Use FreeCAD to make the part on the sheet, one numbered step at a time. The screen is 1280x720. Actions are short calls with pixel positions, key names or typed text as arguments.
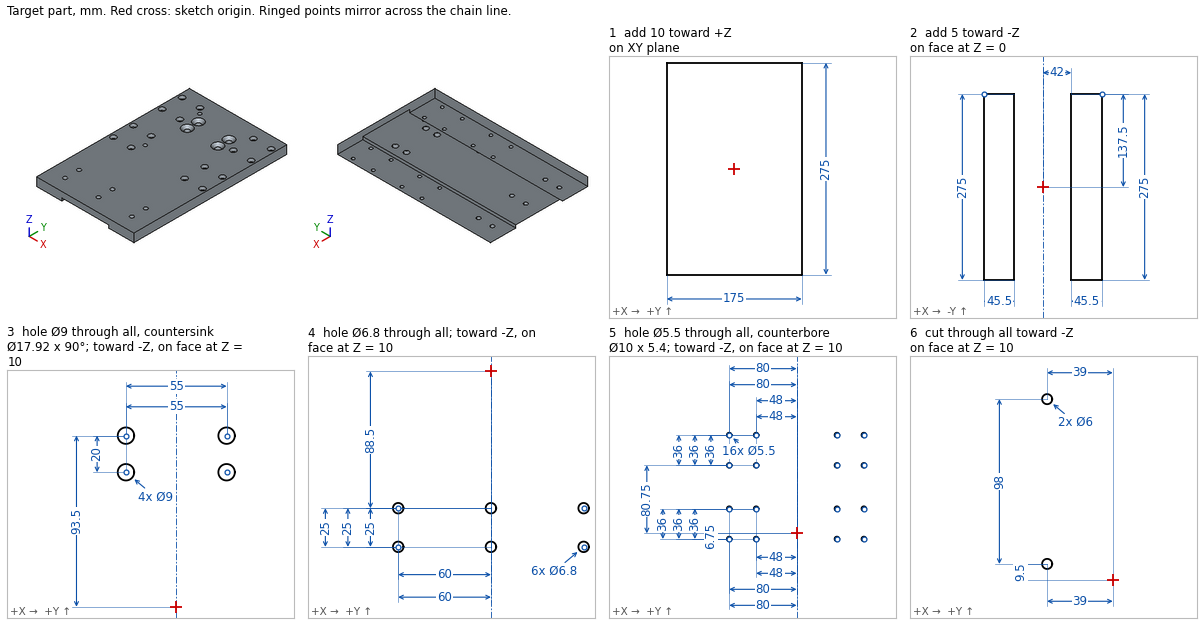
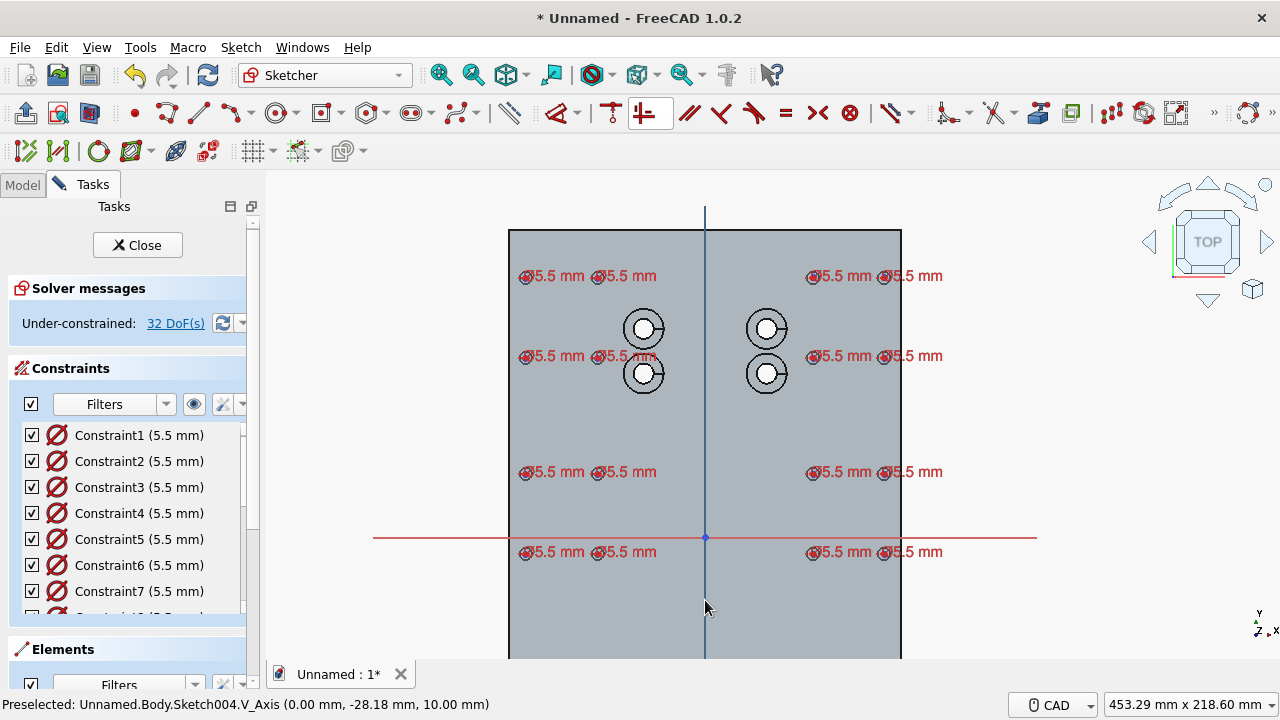
key(s)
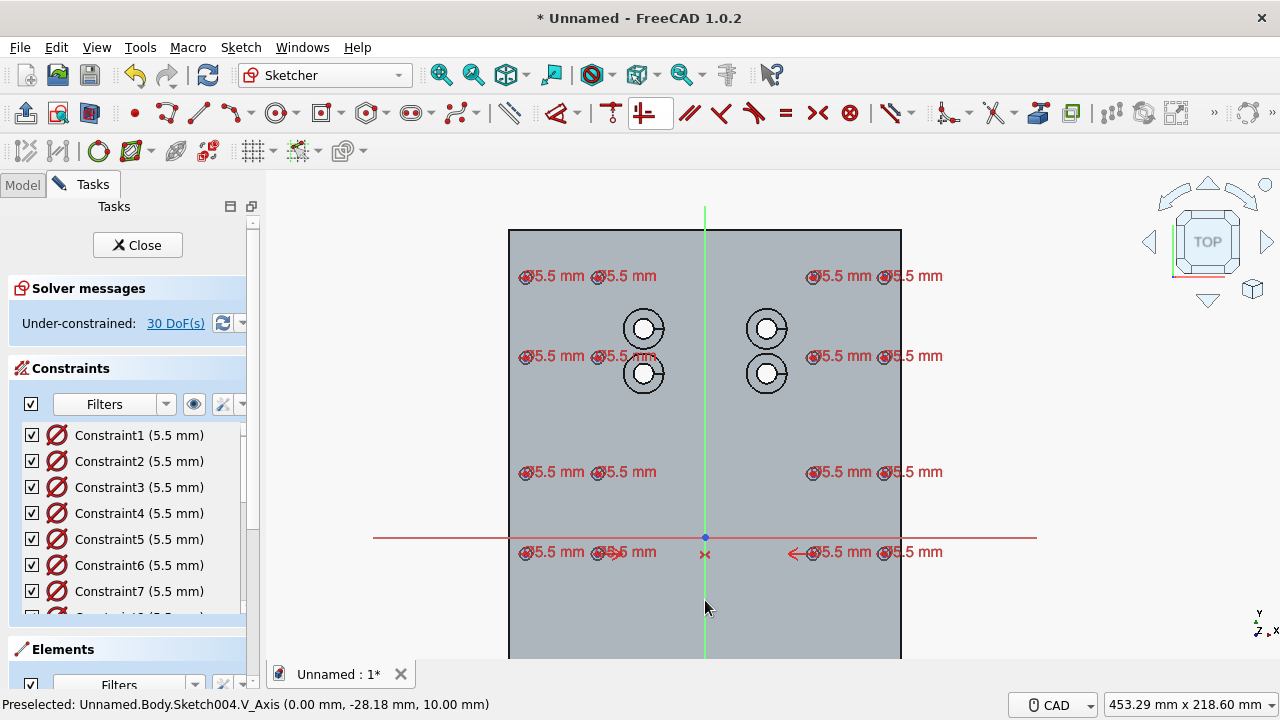
click(526, 554)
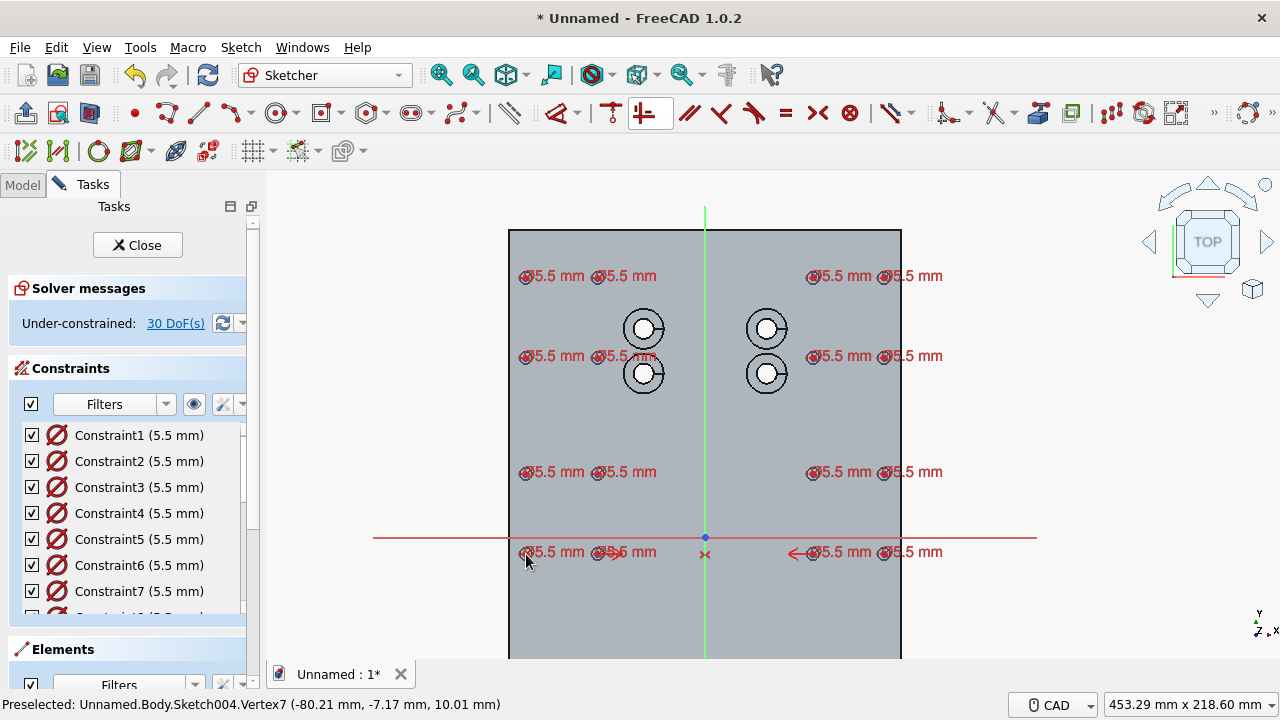
click(884, 554)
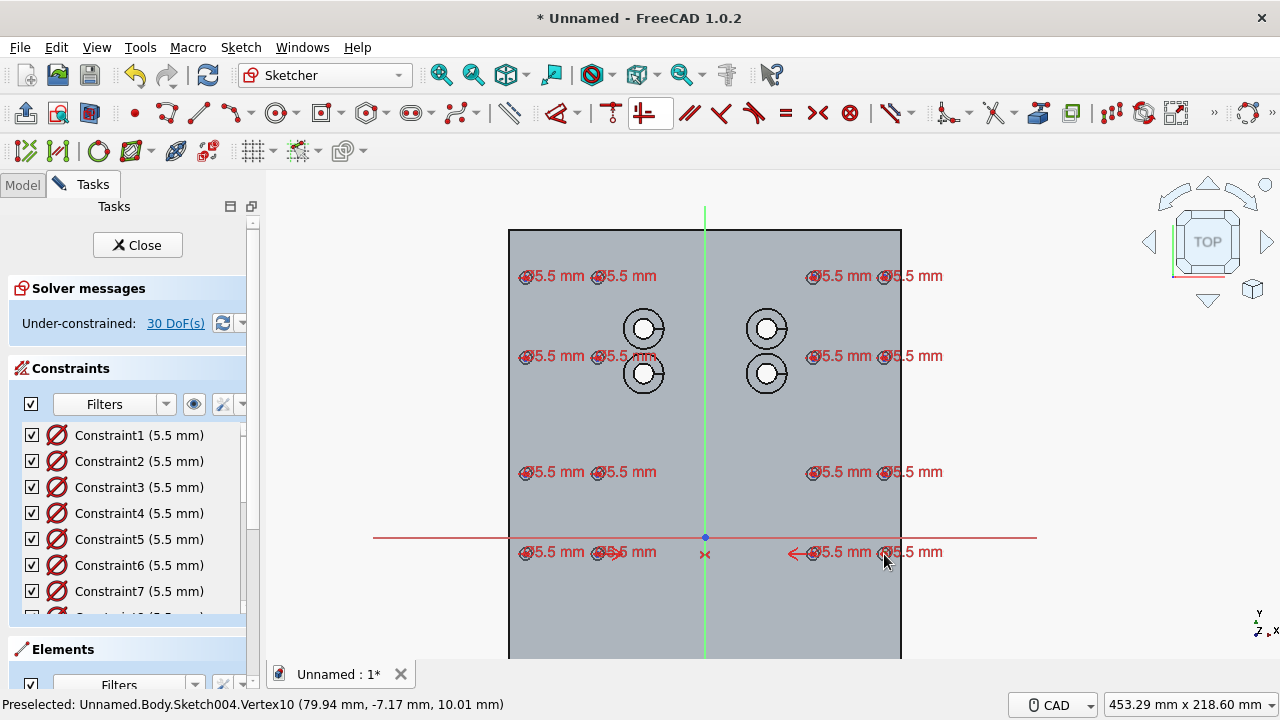
click(705, 600)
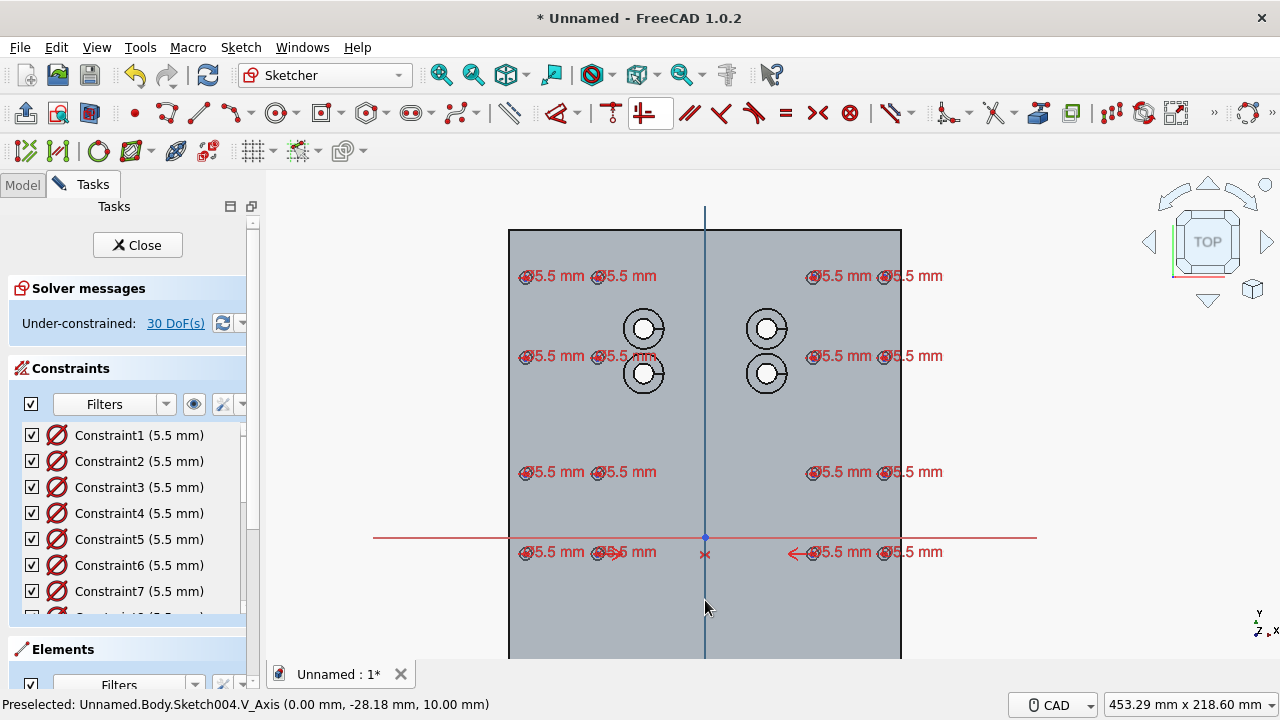
key(s)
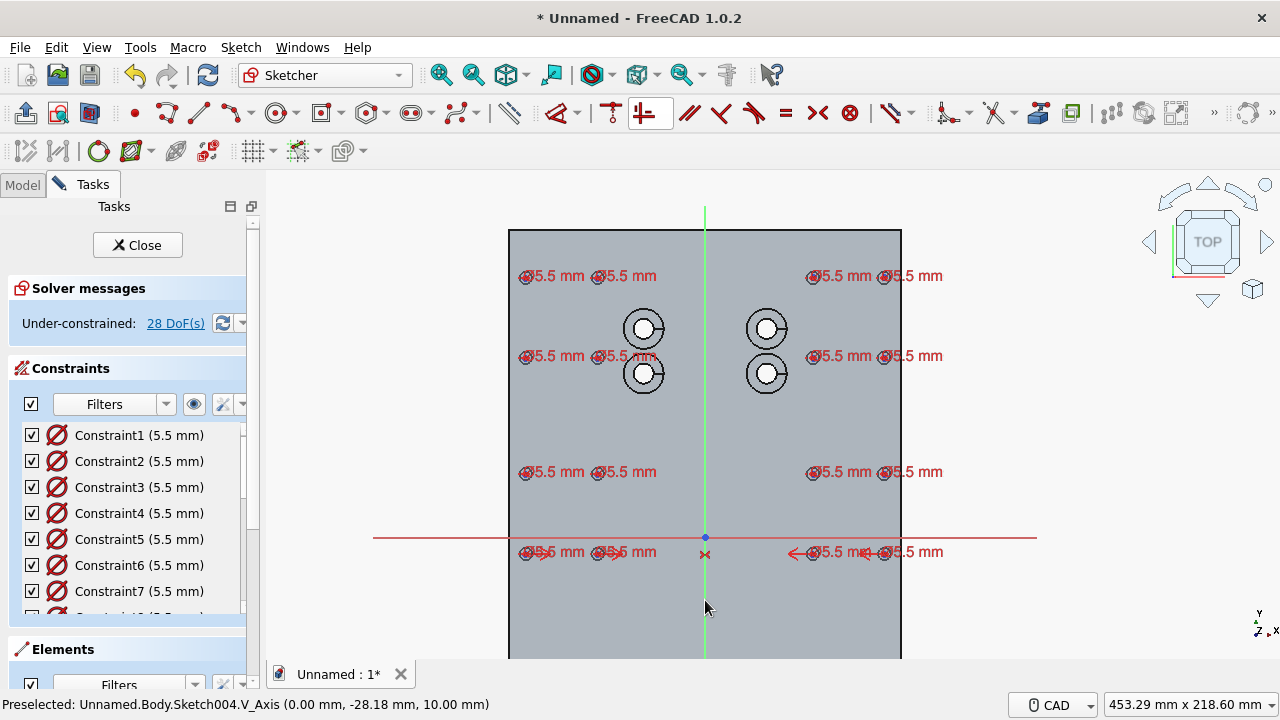
click(598, 474)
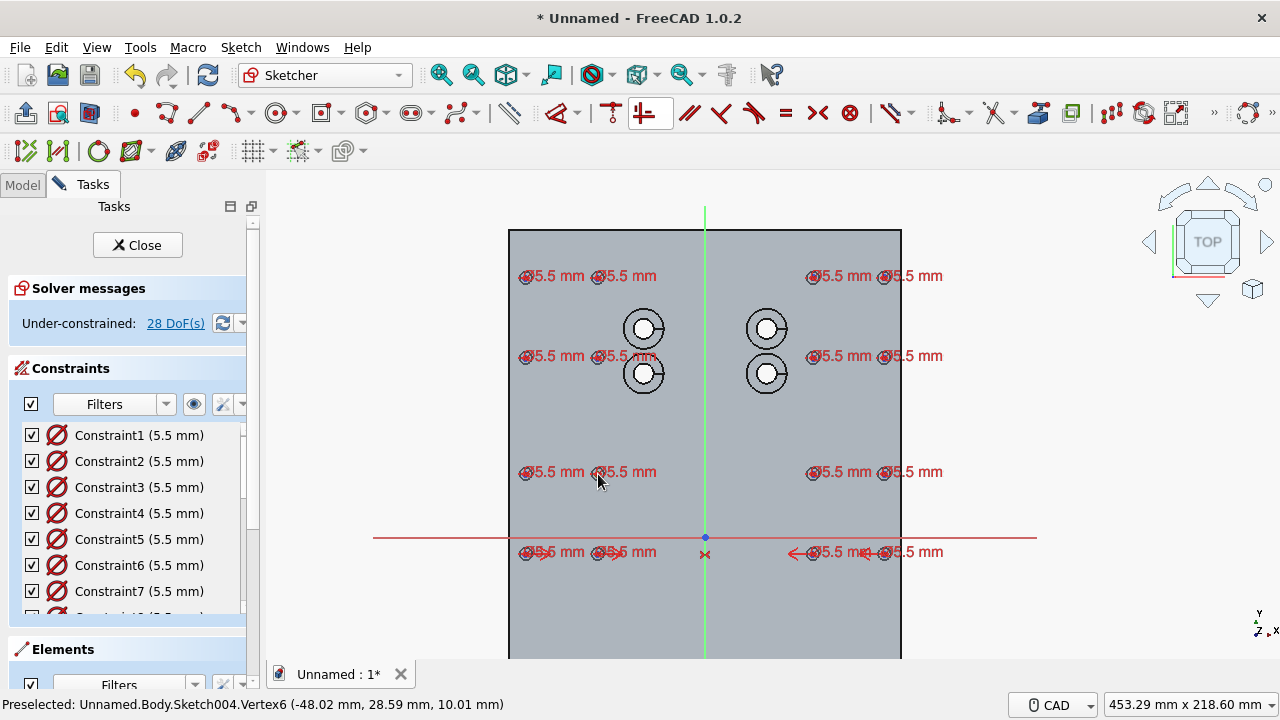
click(813, 474)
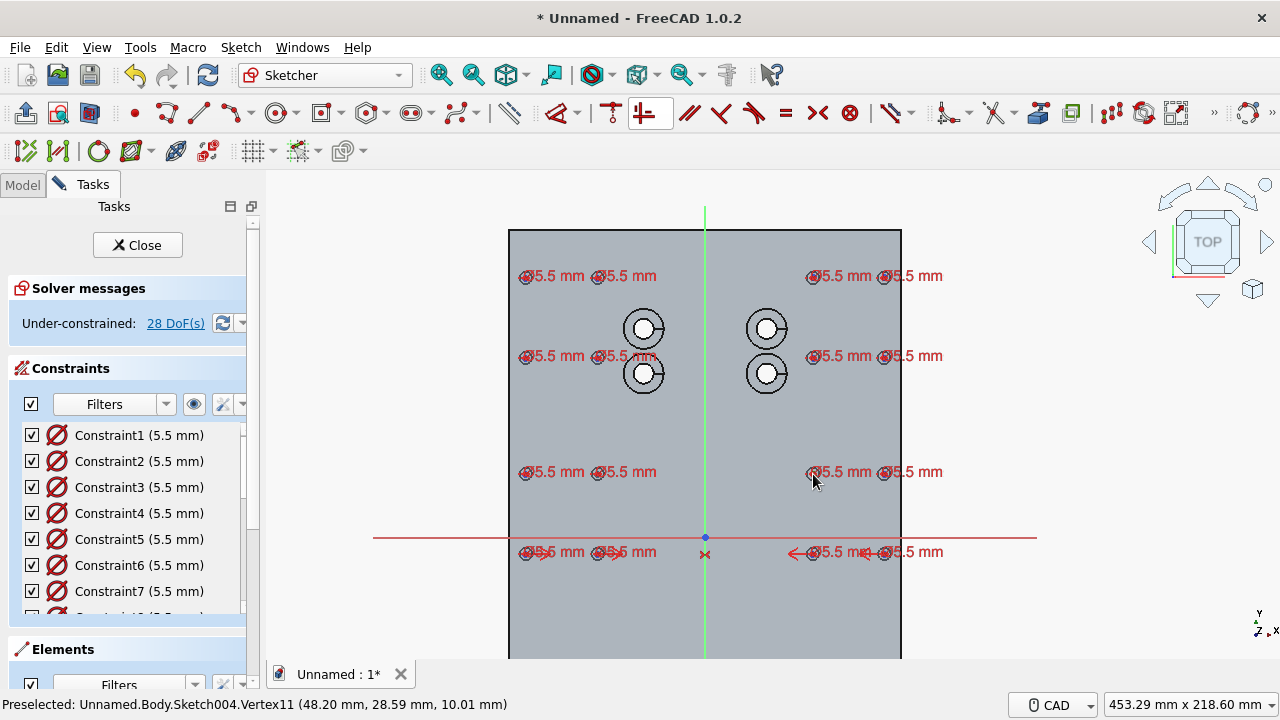
click(705, 600)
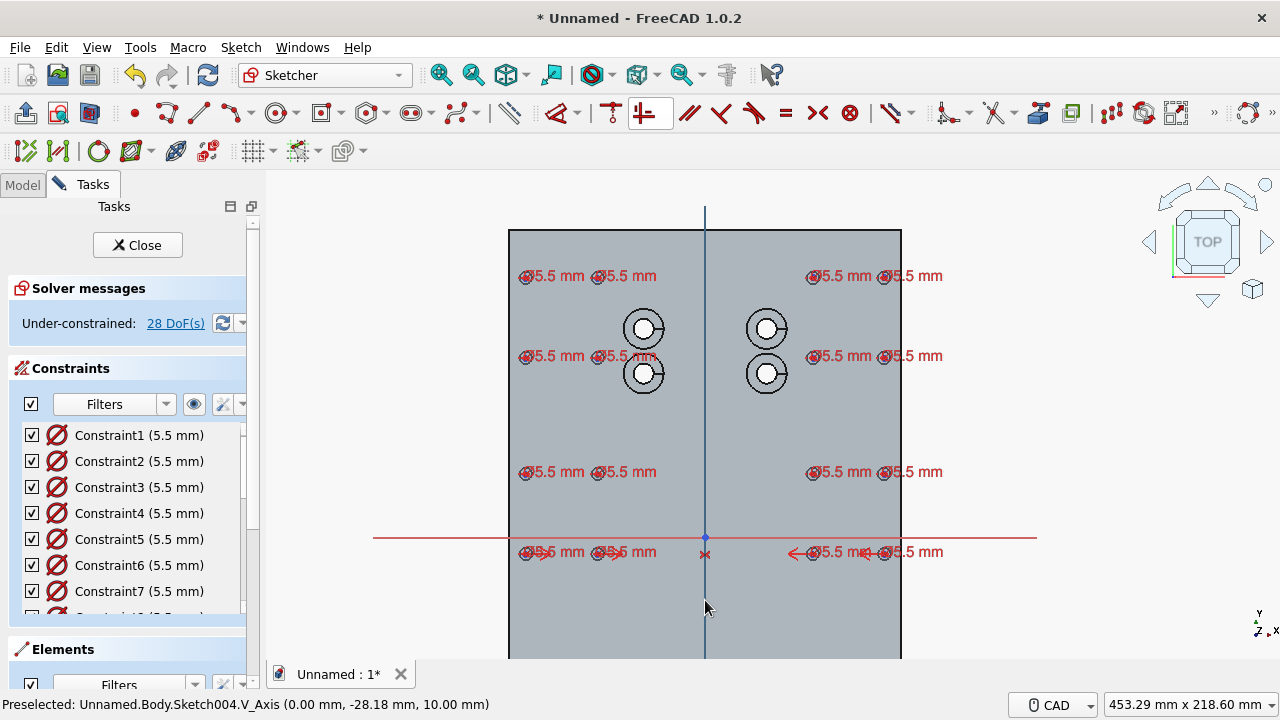
key(s)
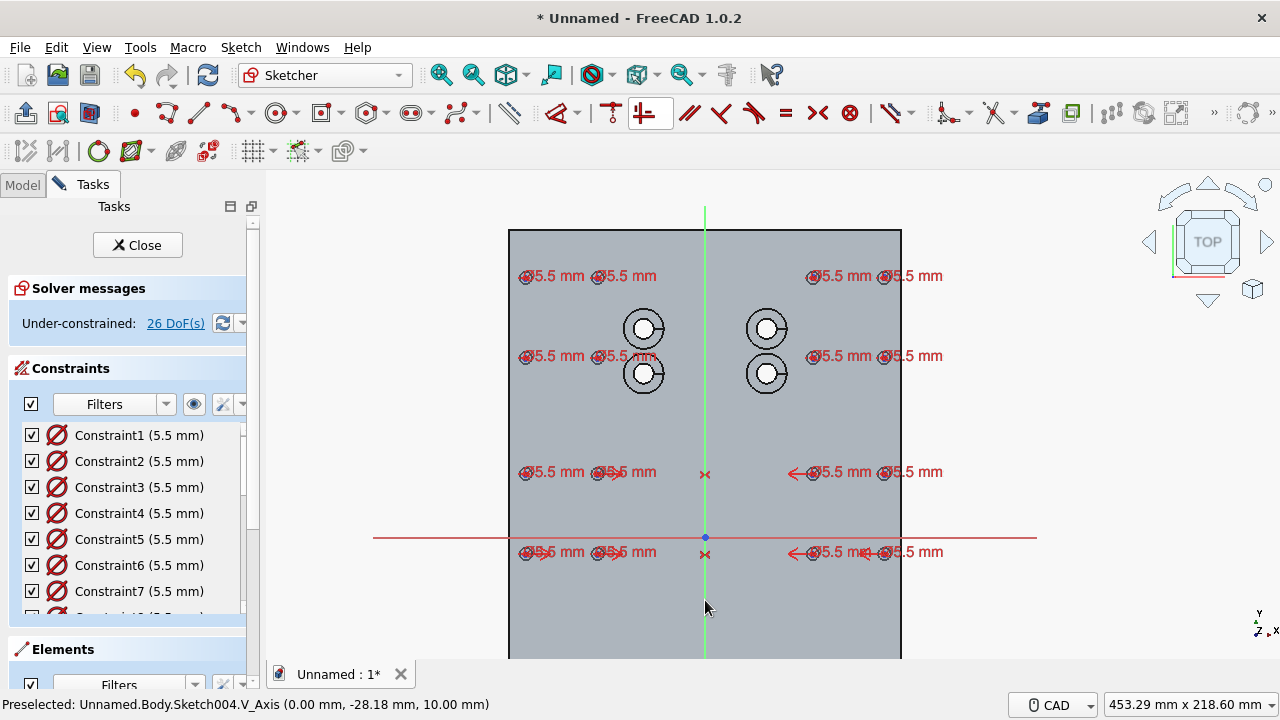
click(526, 474)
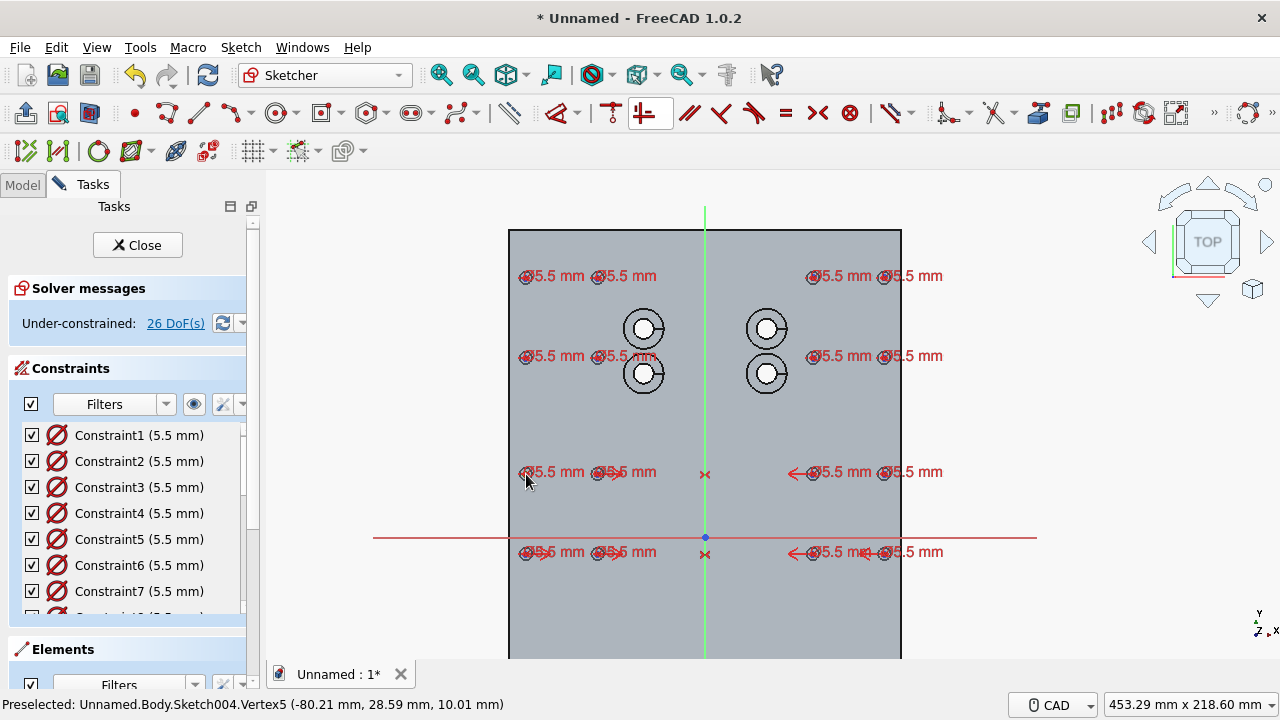
click(884, 474)